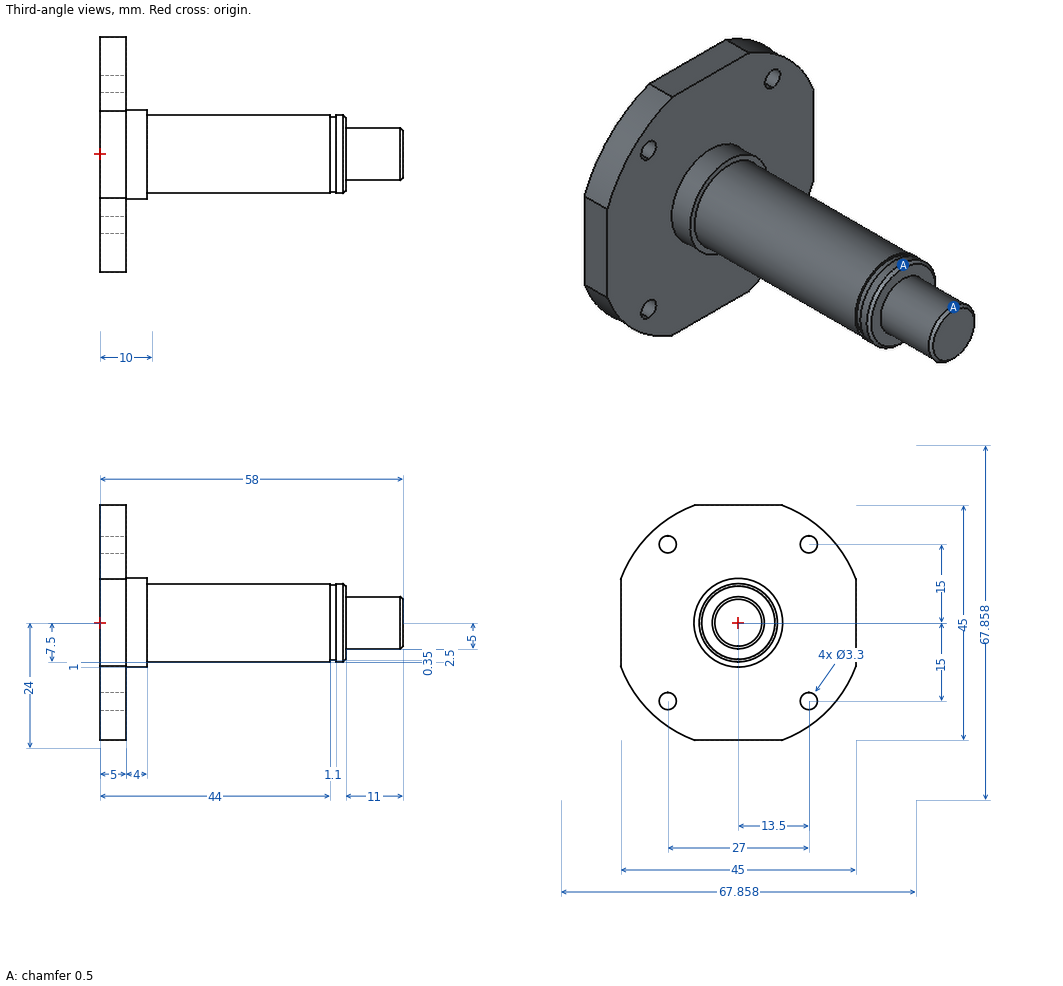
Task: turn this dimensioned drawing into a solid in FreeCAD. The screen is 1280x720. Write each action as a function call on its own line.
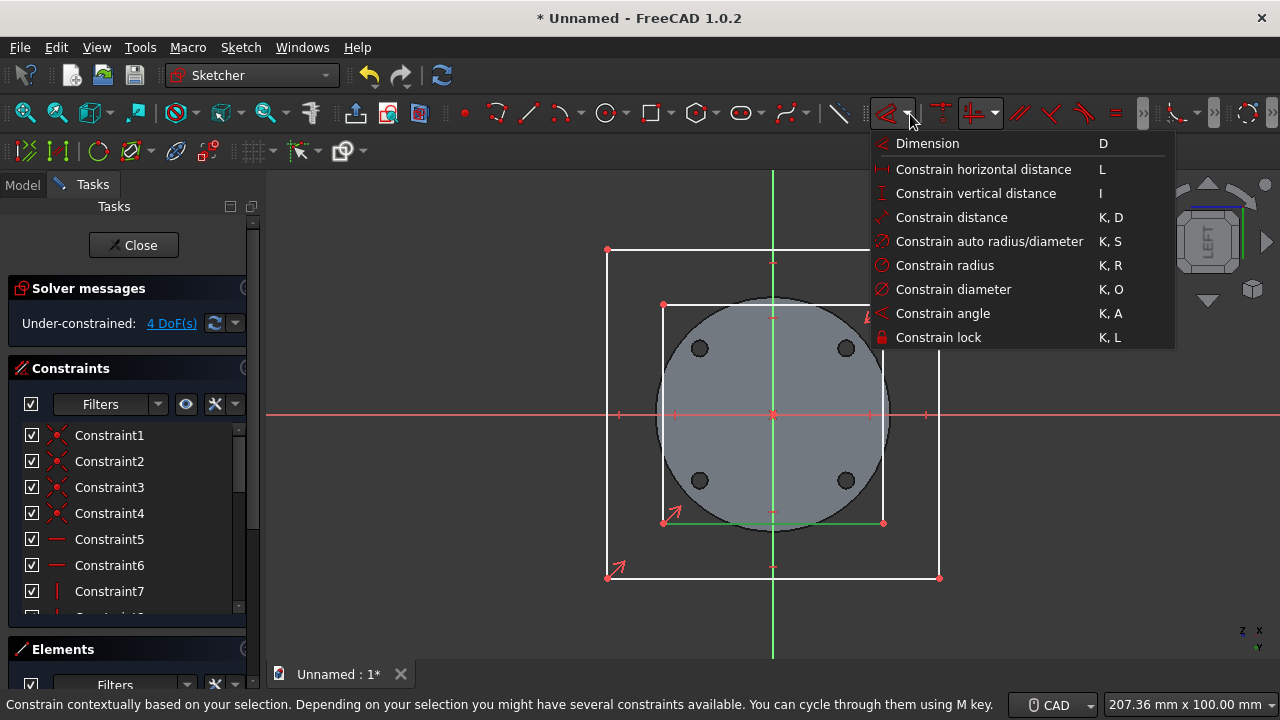
click(1023, 169)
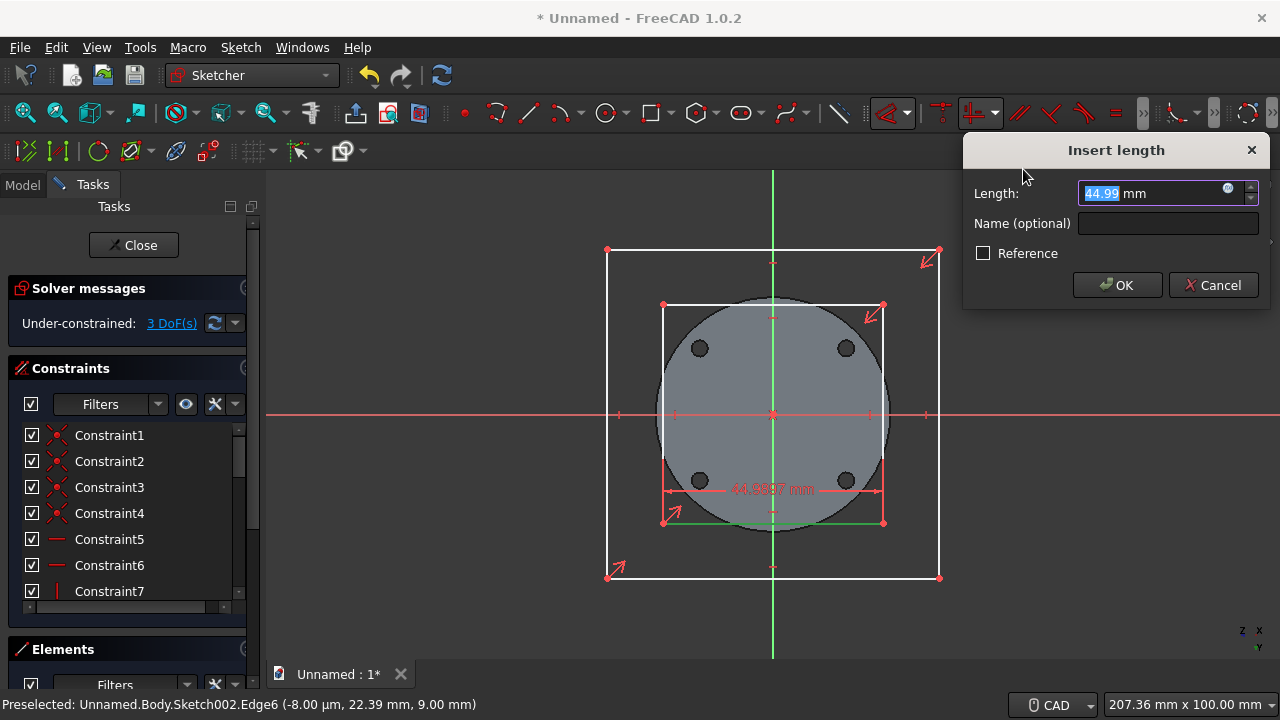
text(45)
key(Return)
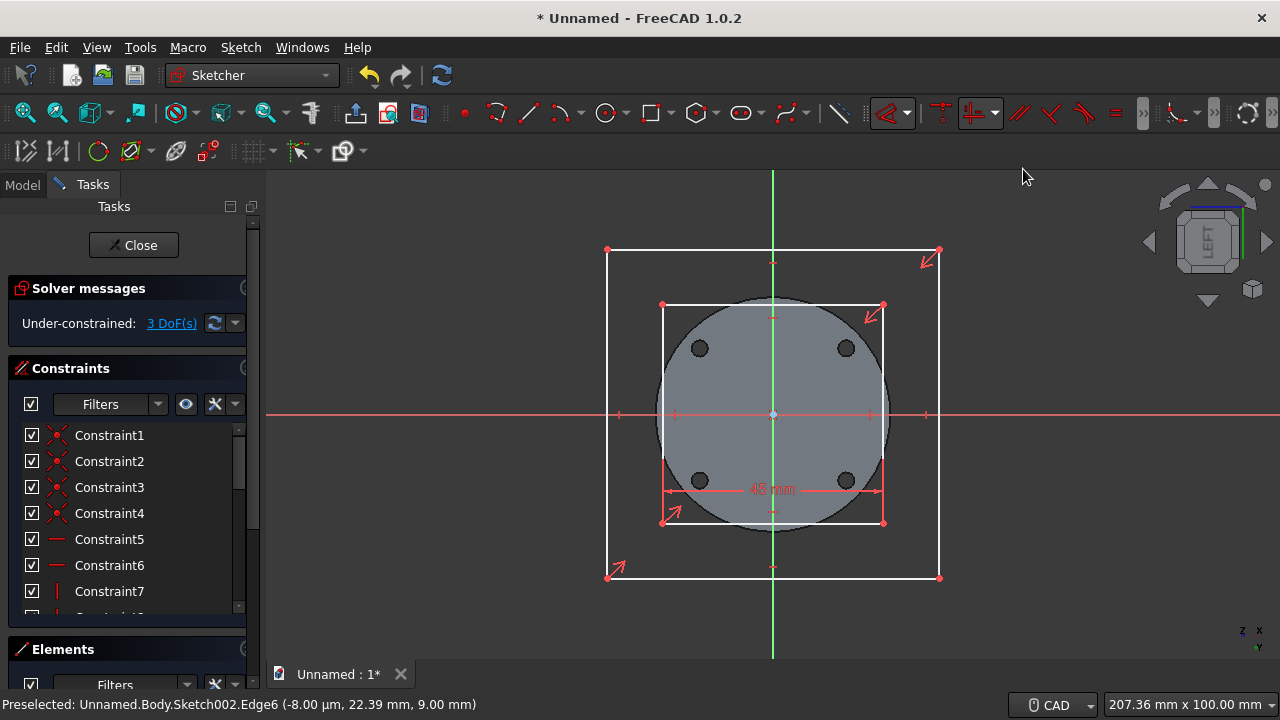
click(883, 458)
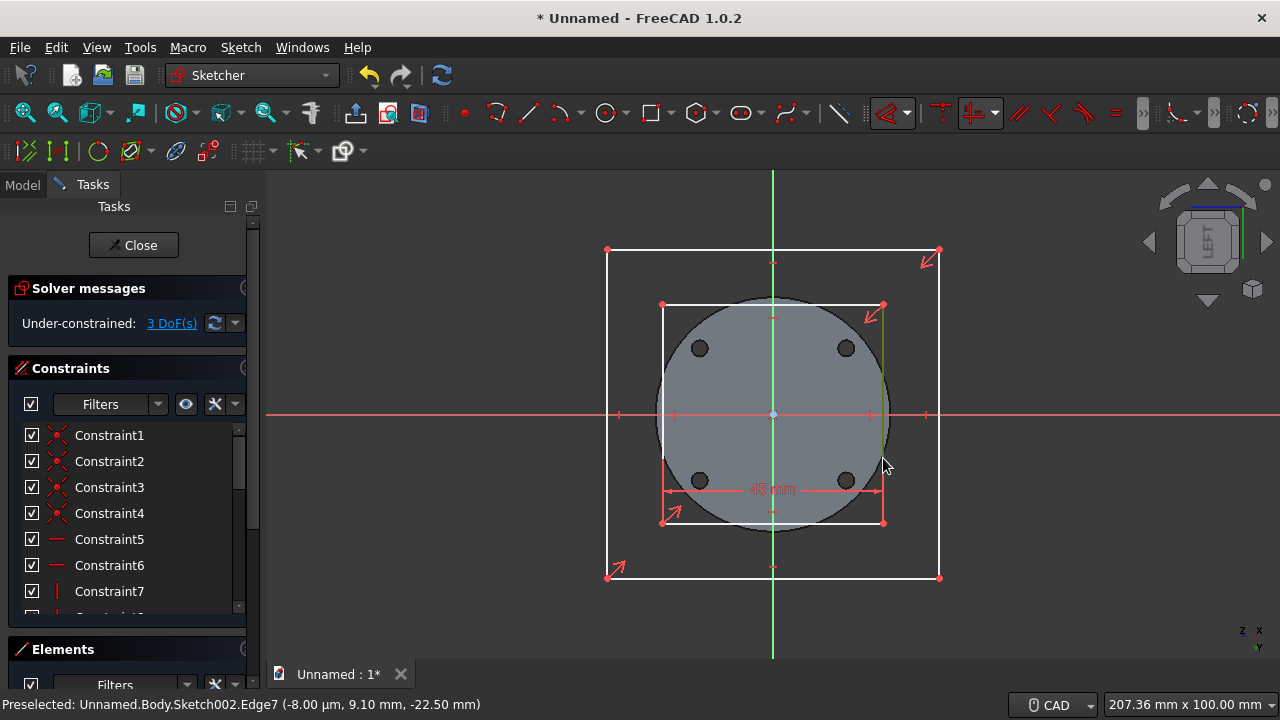
key(i)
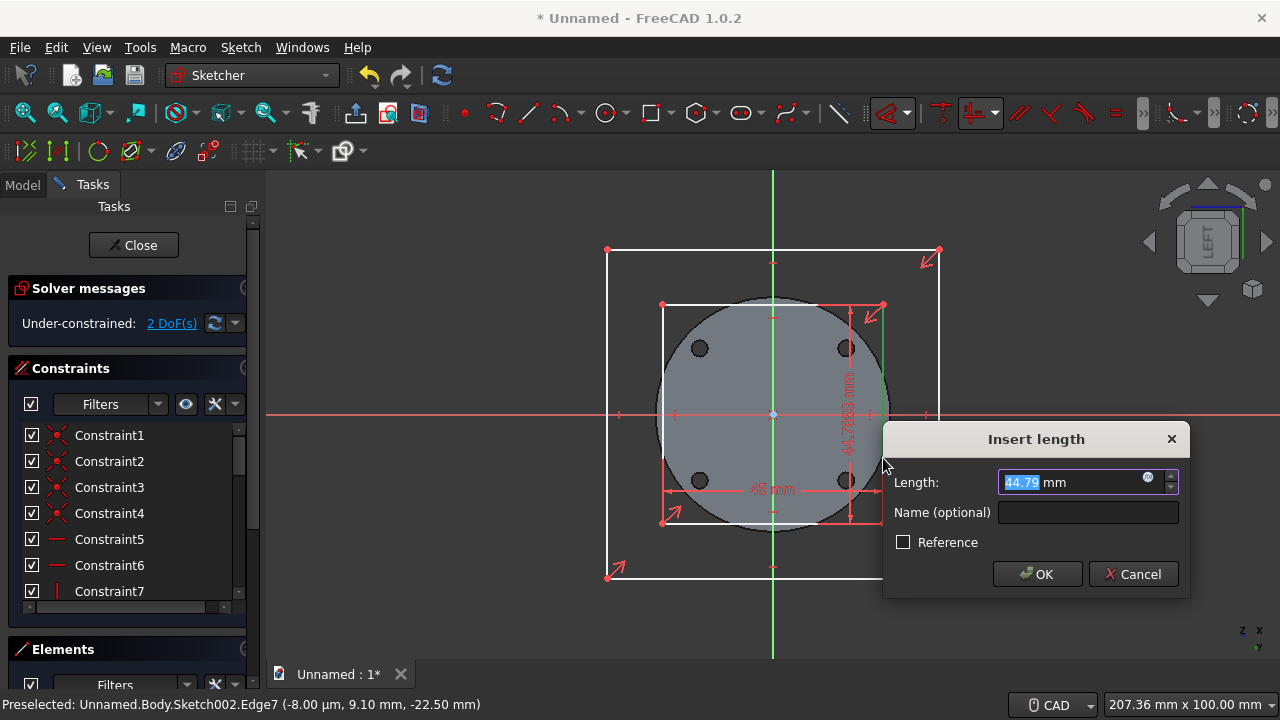
text(45)
key(Return)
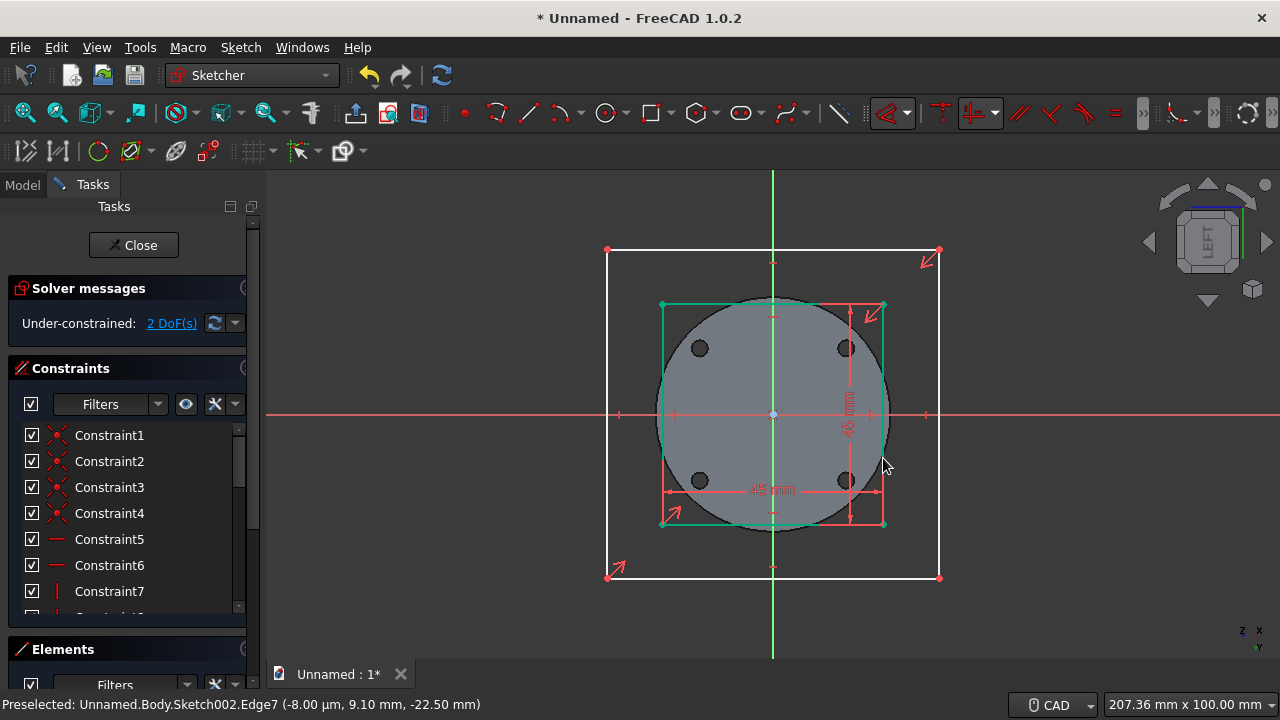
click(707, 579)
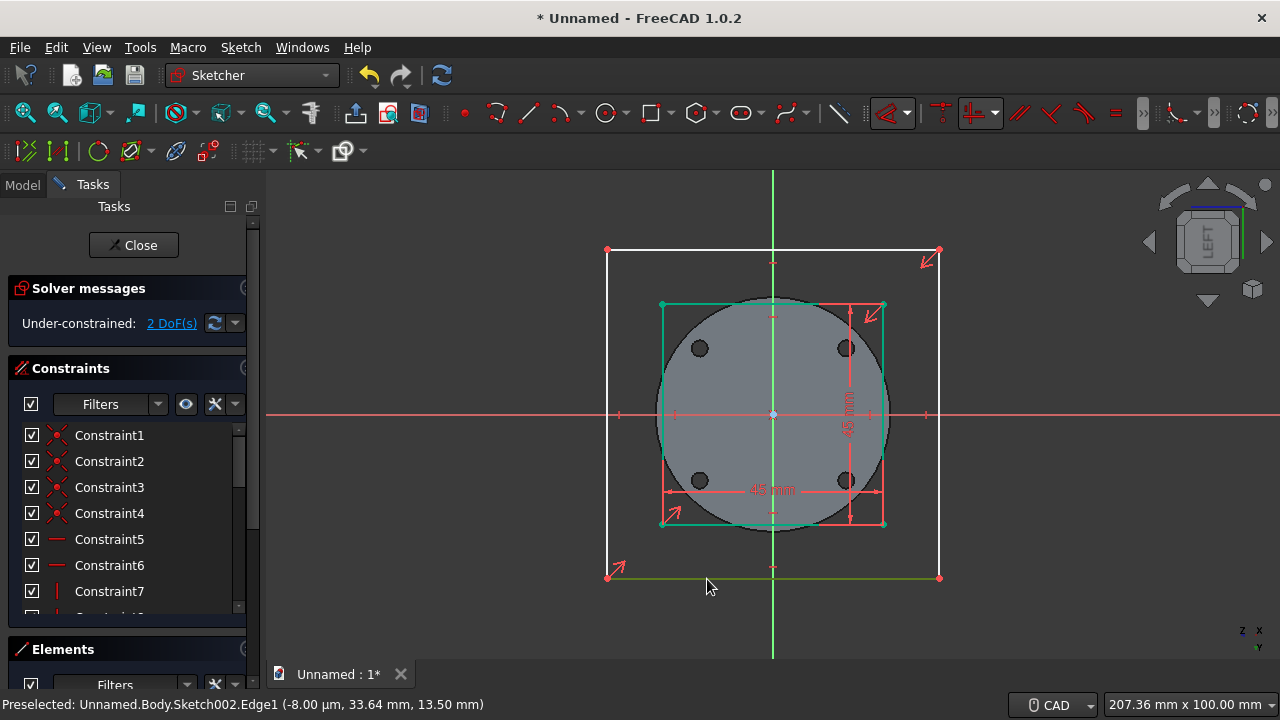
click(910, 114)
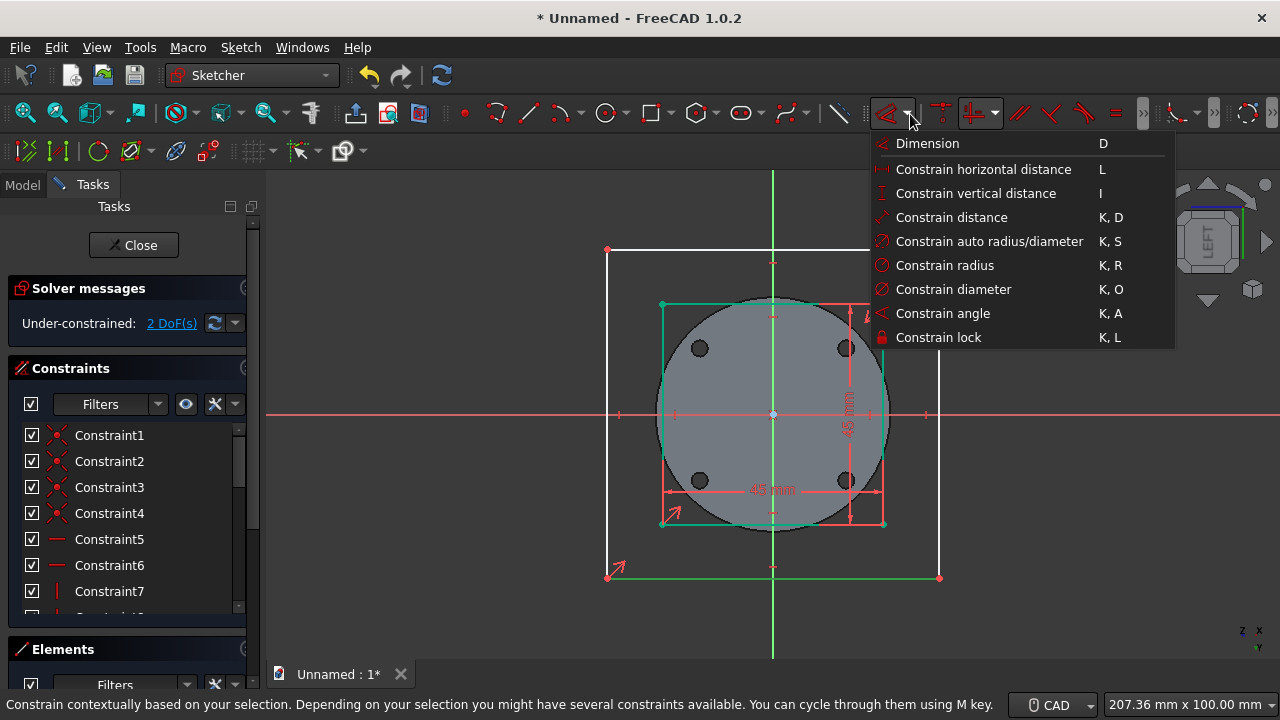
click(1023, 169)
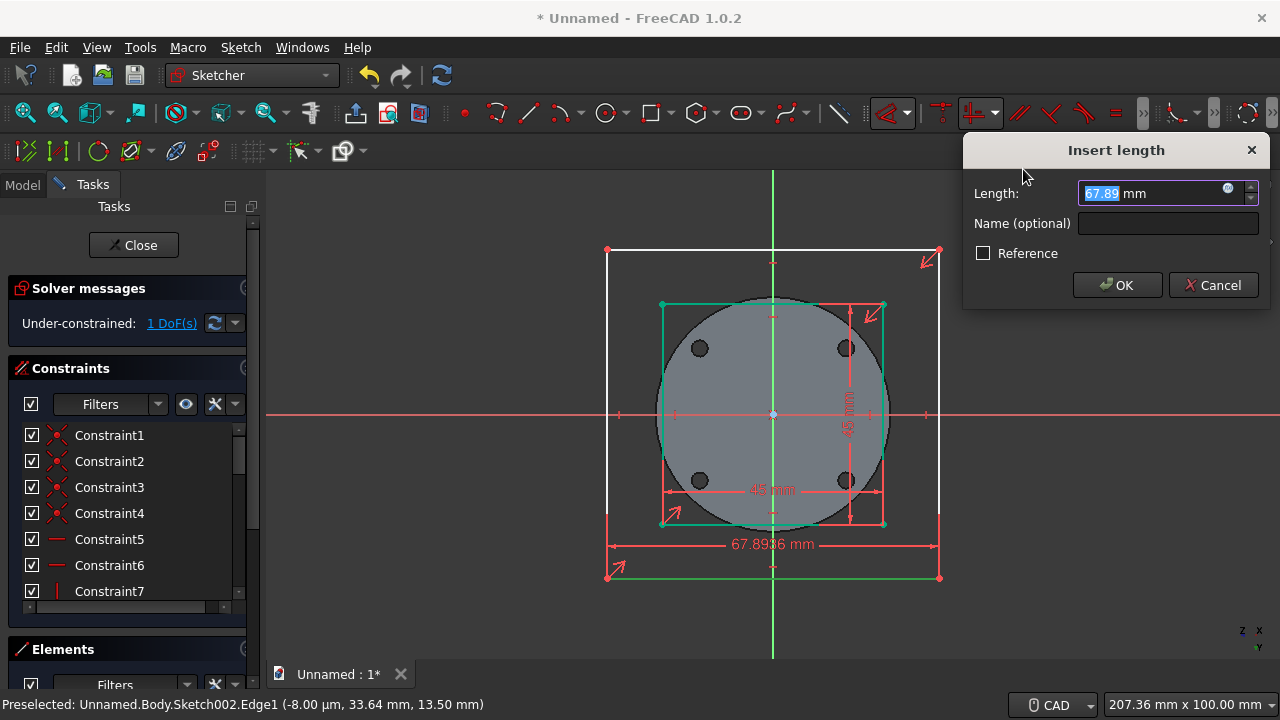
text(67.858)
key(Return)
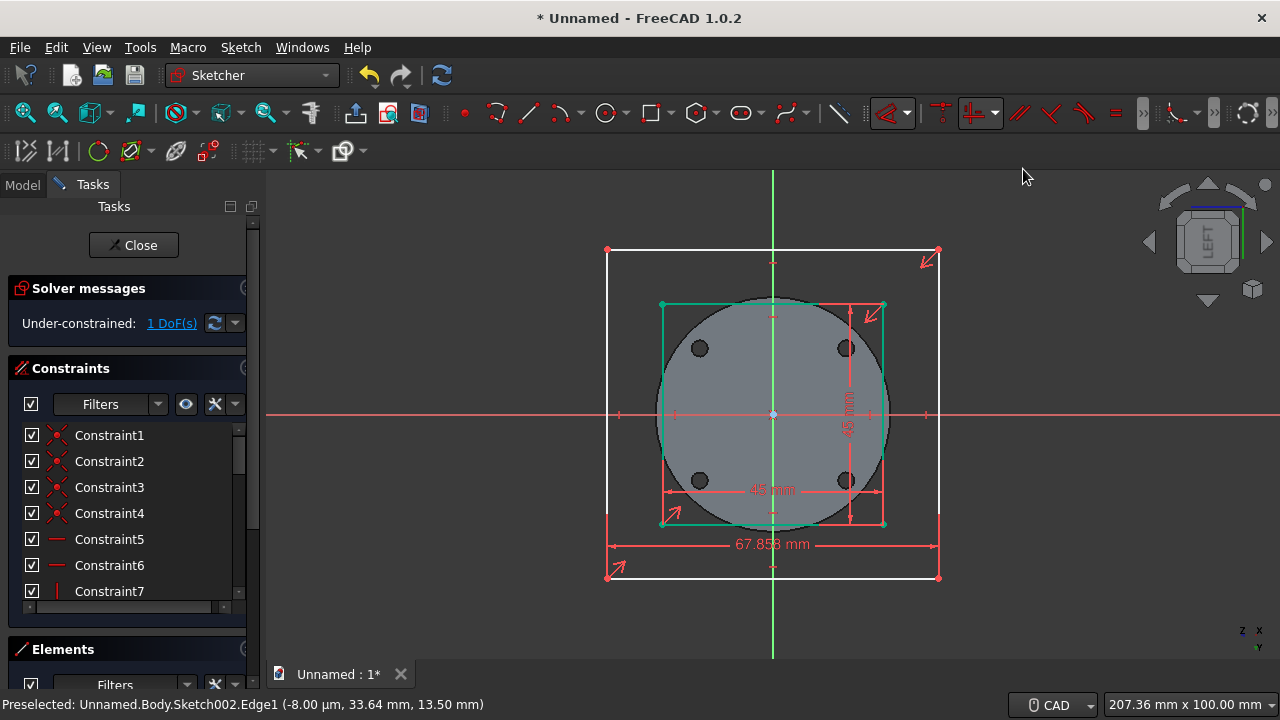
click(939, 480)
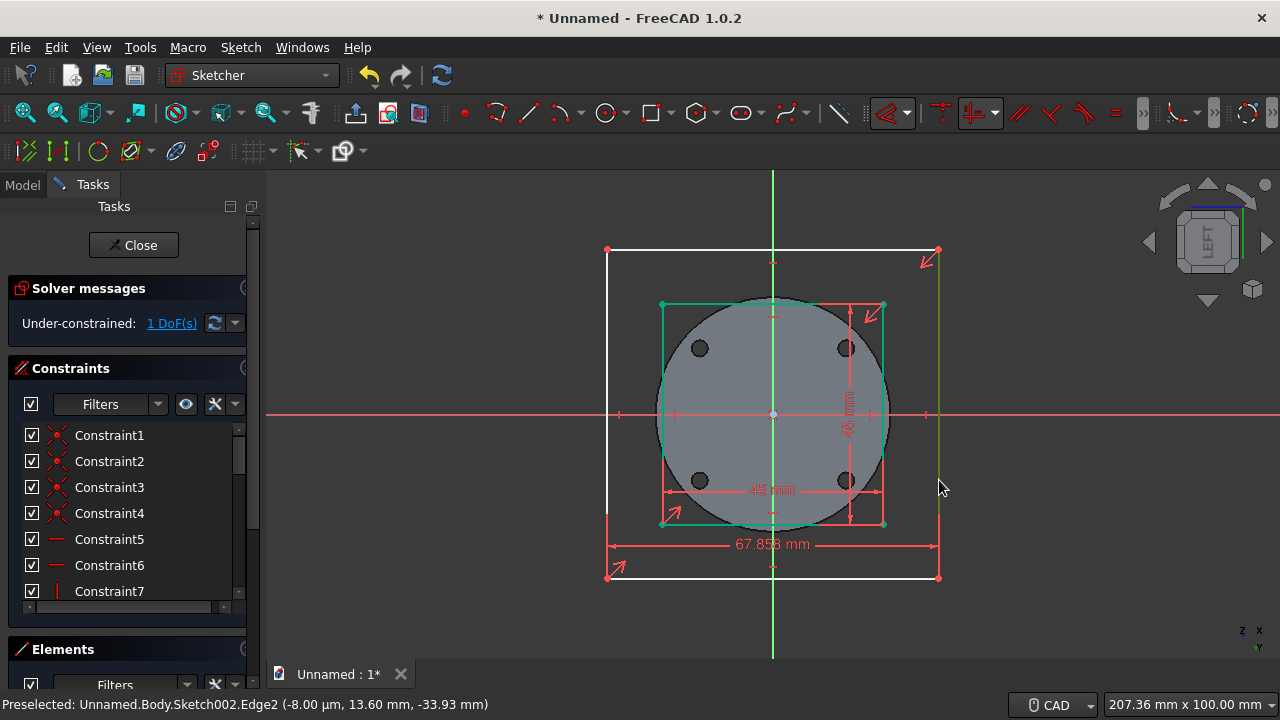
click(910, 114)